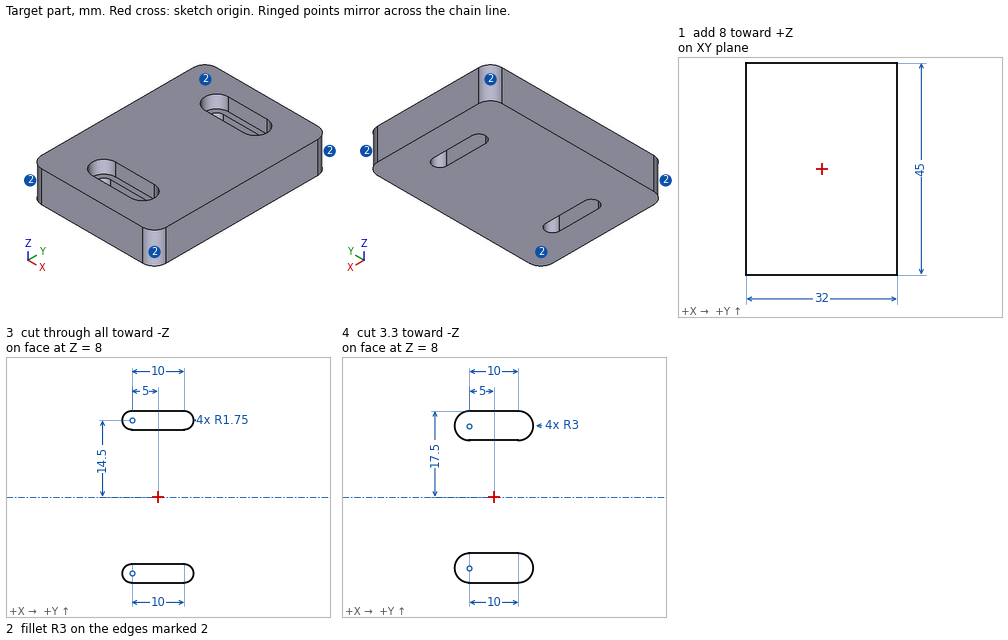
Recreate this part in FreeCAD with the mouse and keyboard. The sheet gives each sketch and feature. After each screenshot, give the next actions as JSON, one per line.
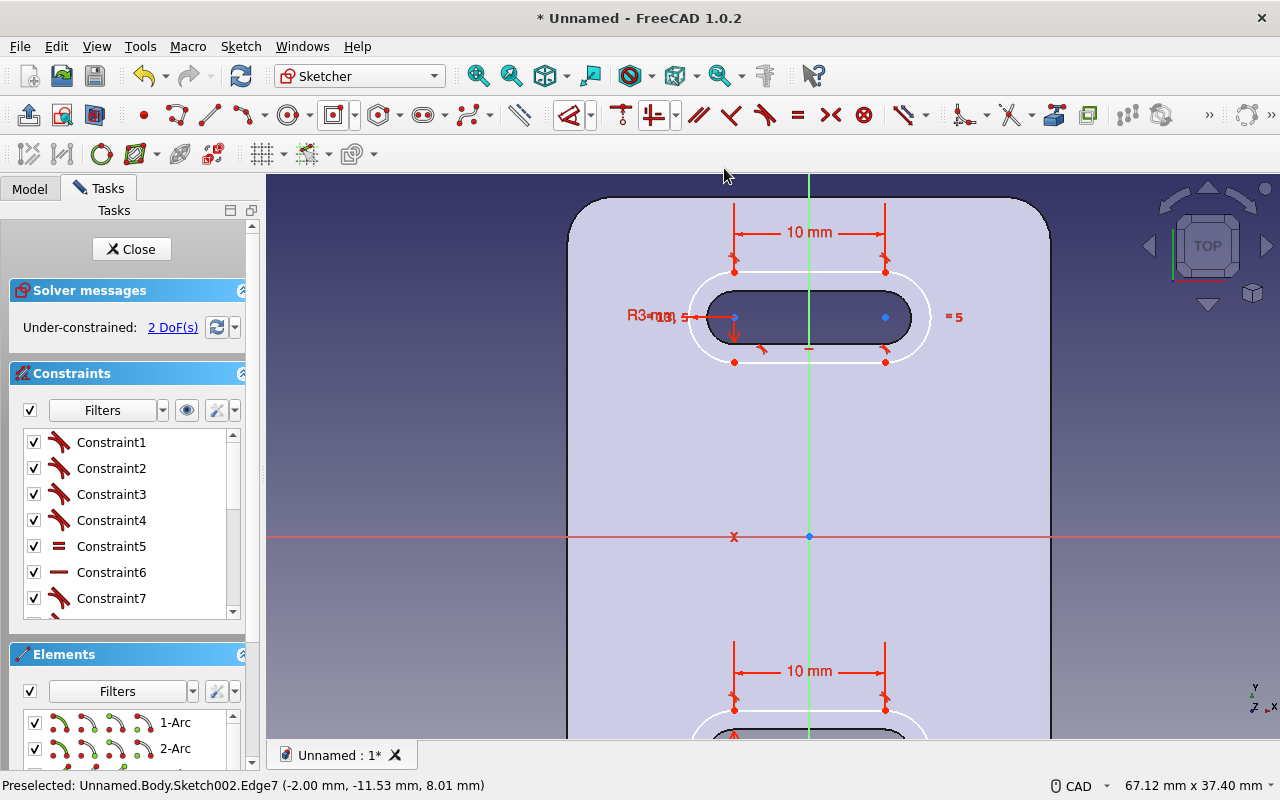
{"action": "left_click", "coordinate": [734, 272]}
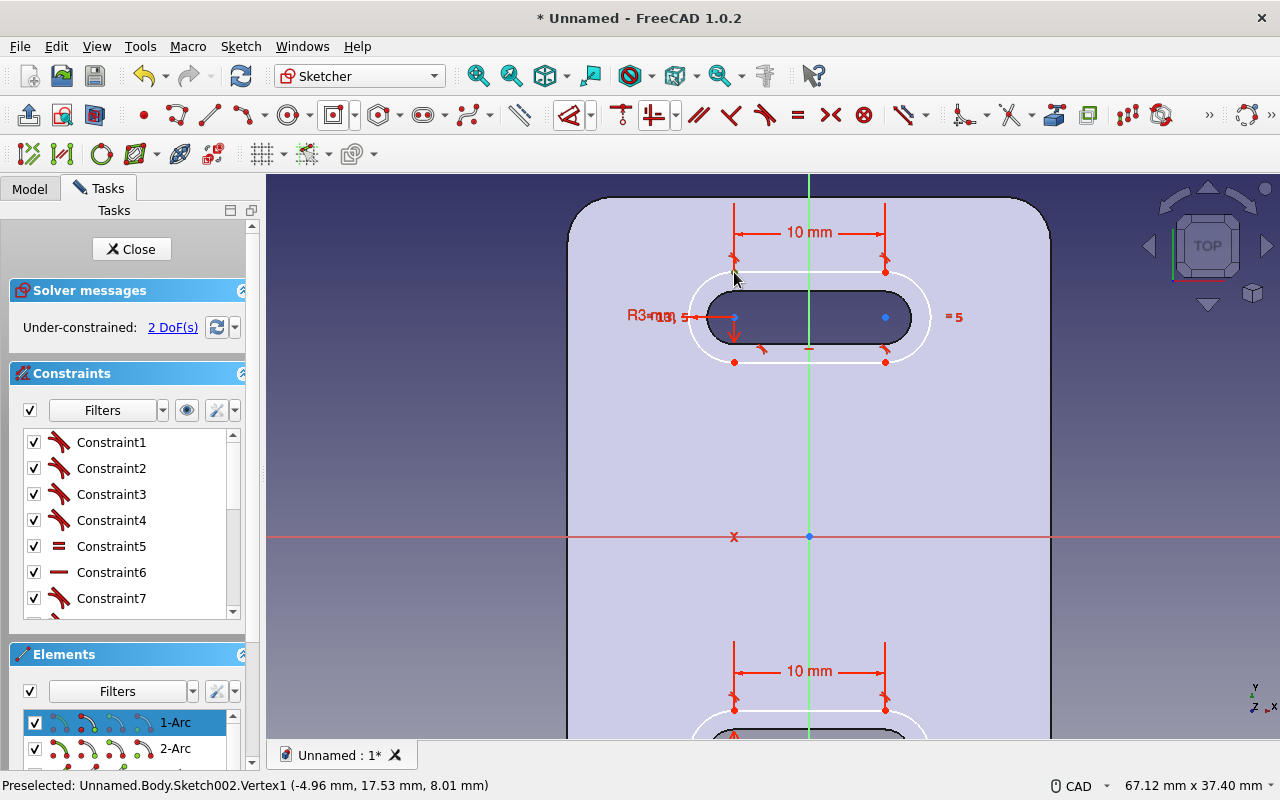
{"action": "key", "text": "l"}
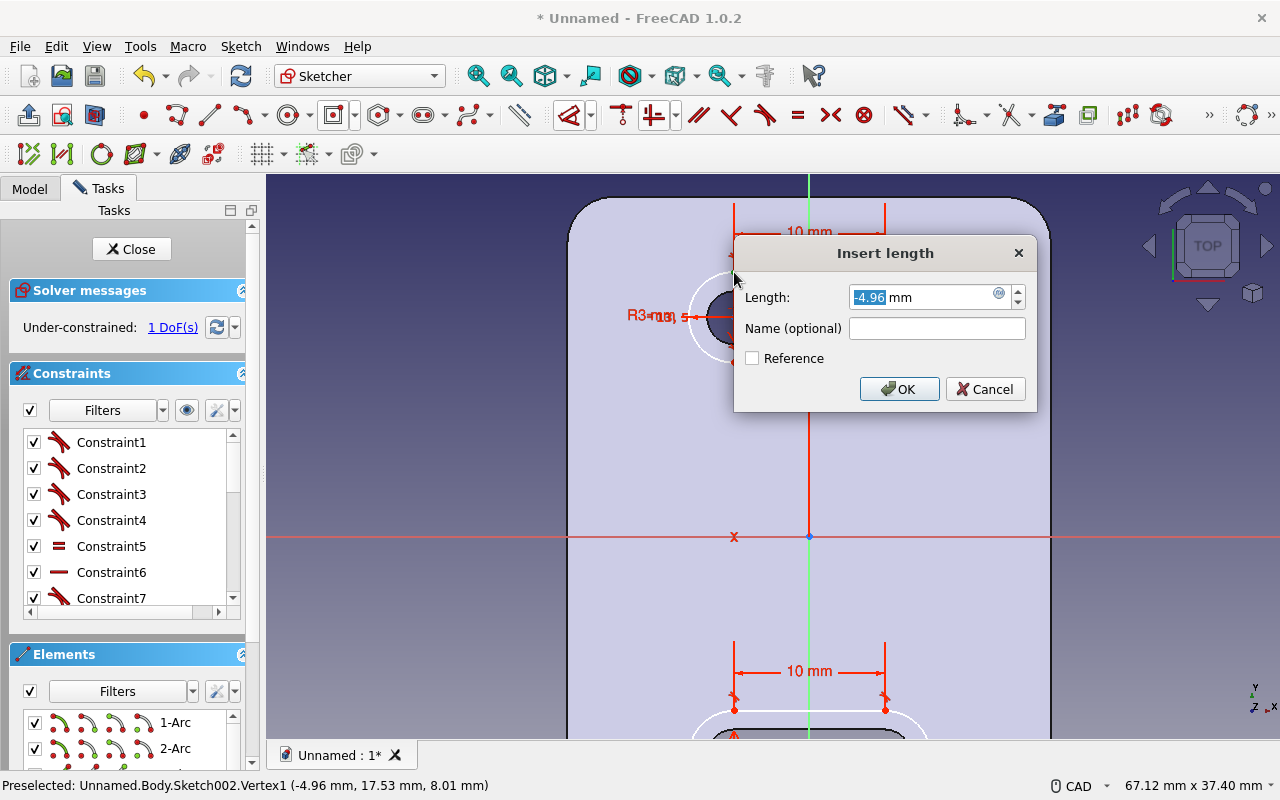
{"action": "type", "text": "-5"}
{"action": "key", "text": "Return"}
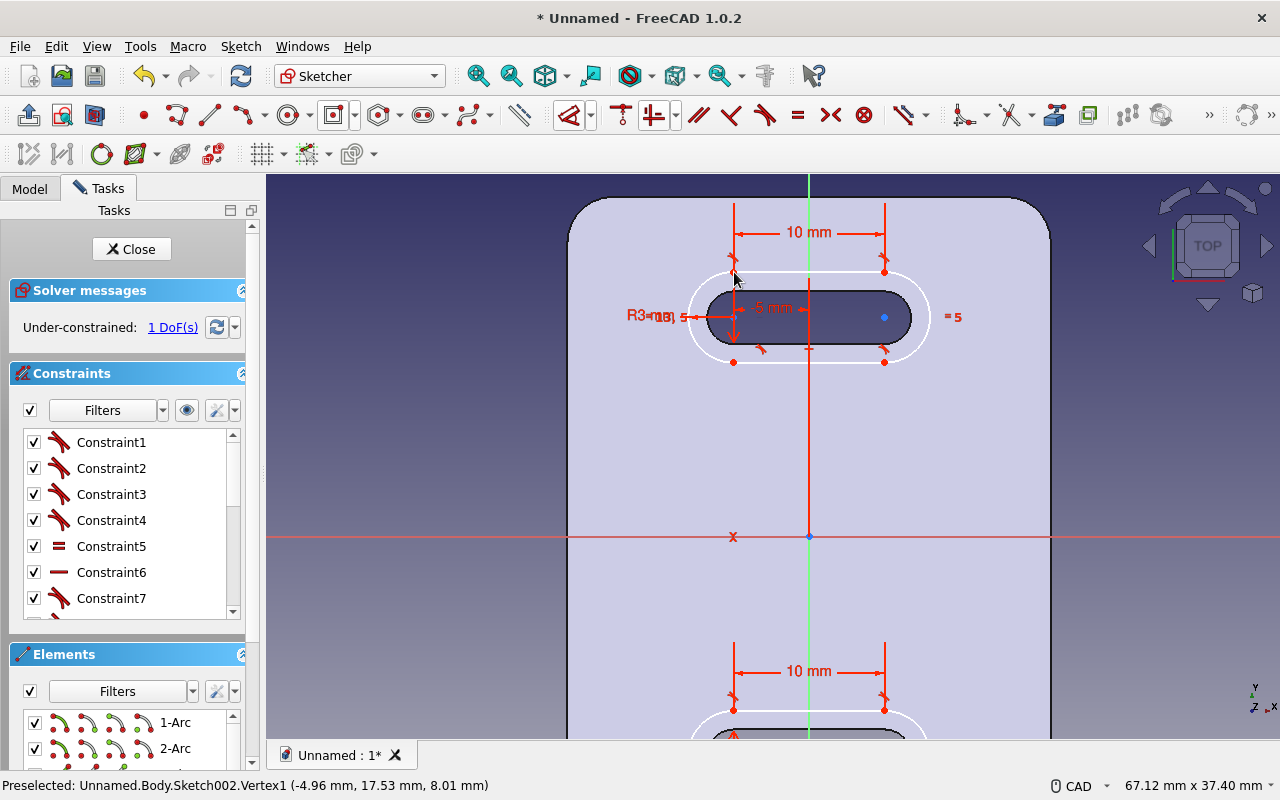
{"action": "left_click", "coordinate": [734, 272]}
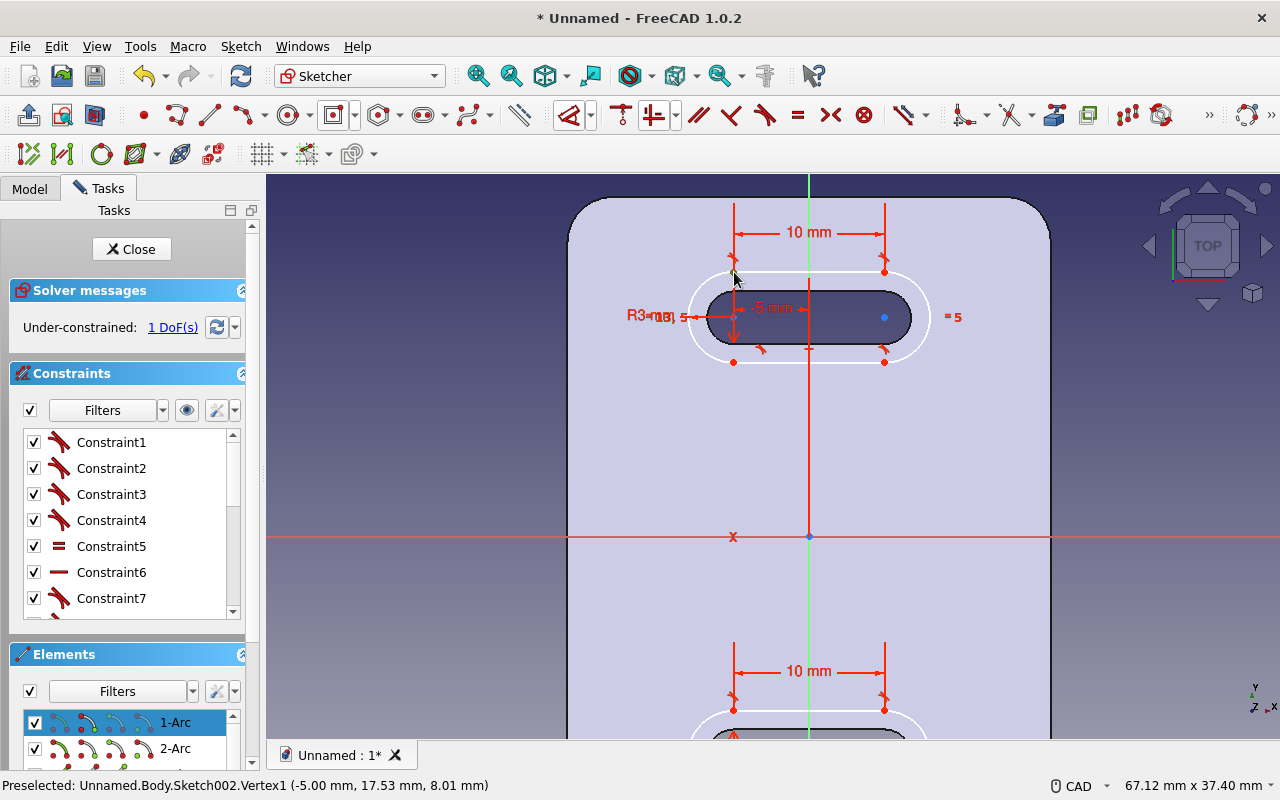
{"action": "key", "text": "i"}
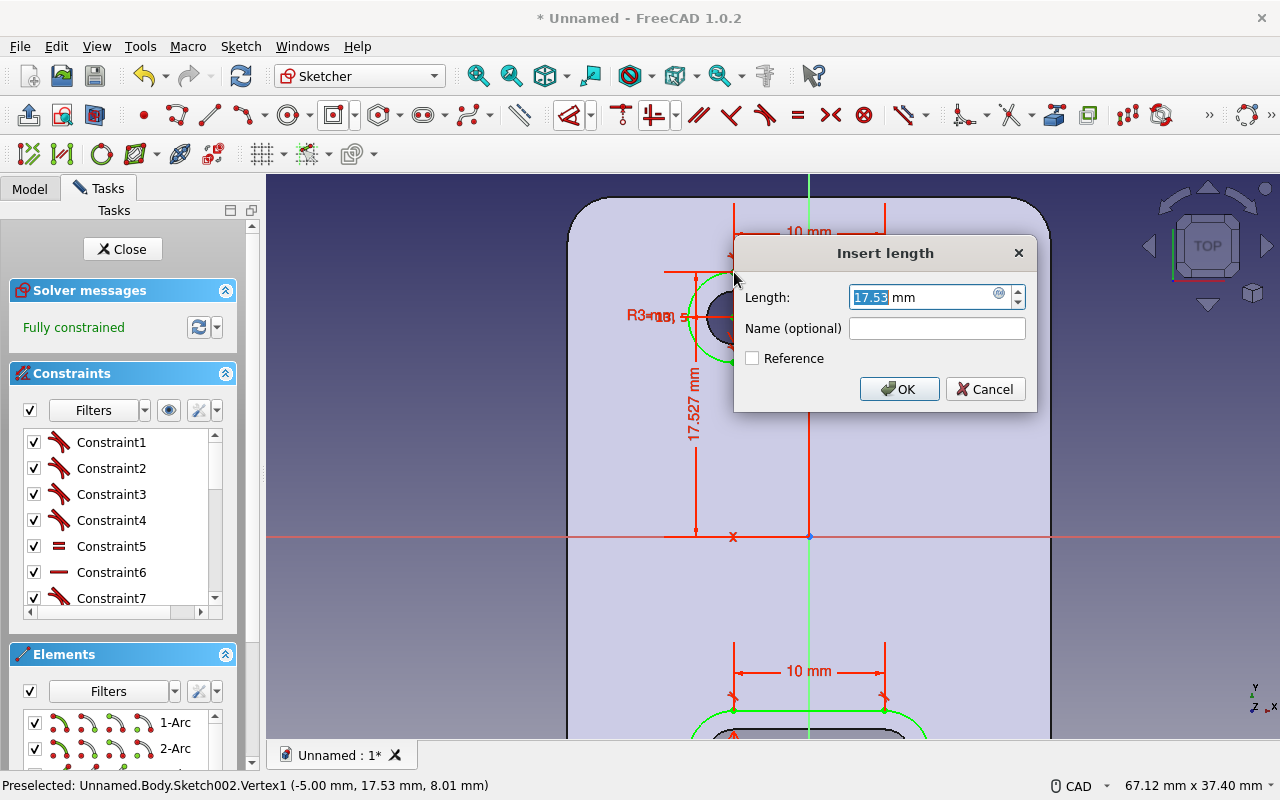
{"action": "type", "text": "17.5"}
{"action": "key", "text": "Return"}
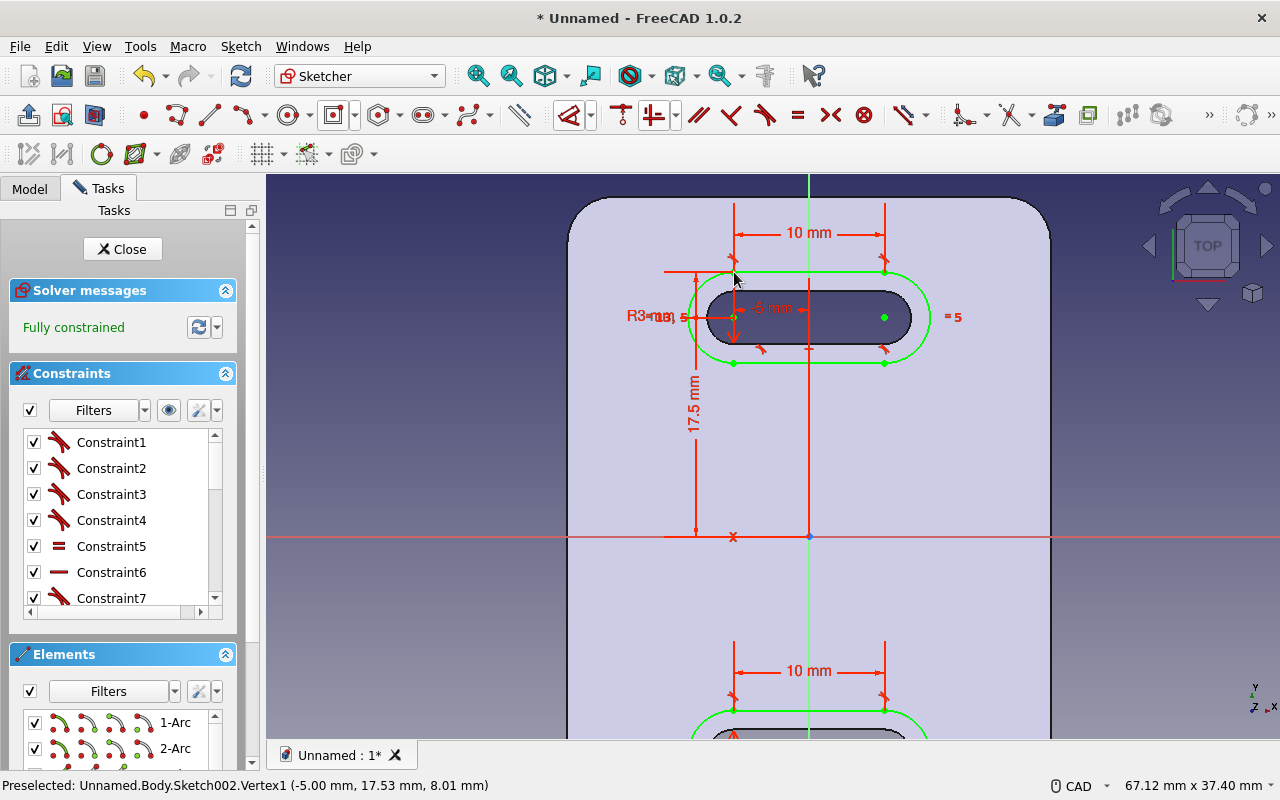
{"action": "left_click", "coordinate": [123, 249]}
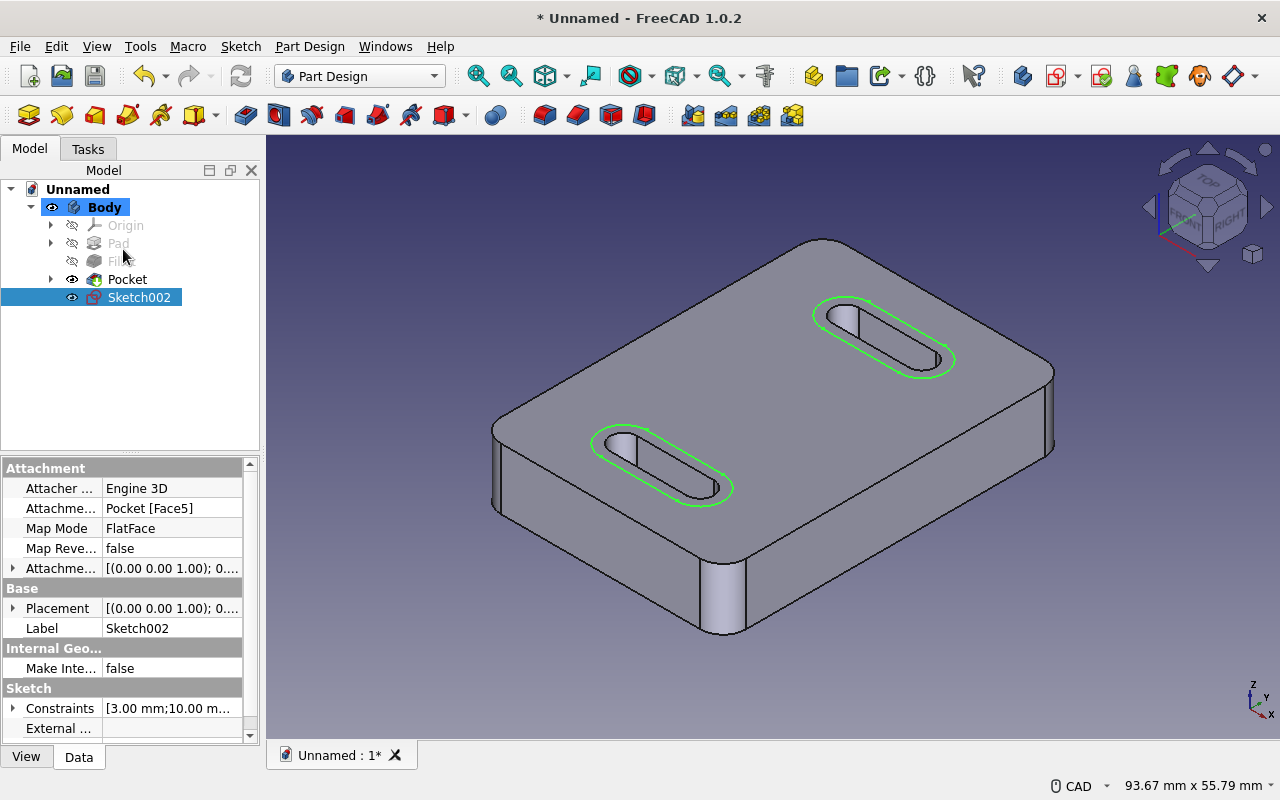
{"action": "left_click", "coordinate": [246, 116]}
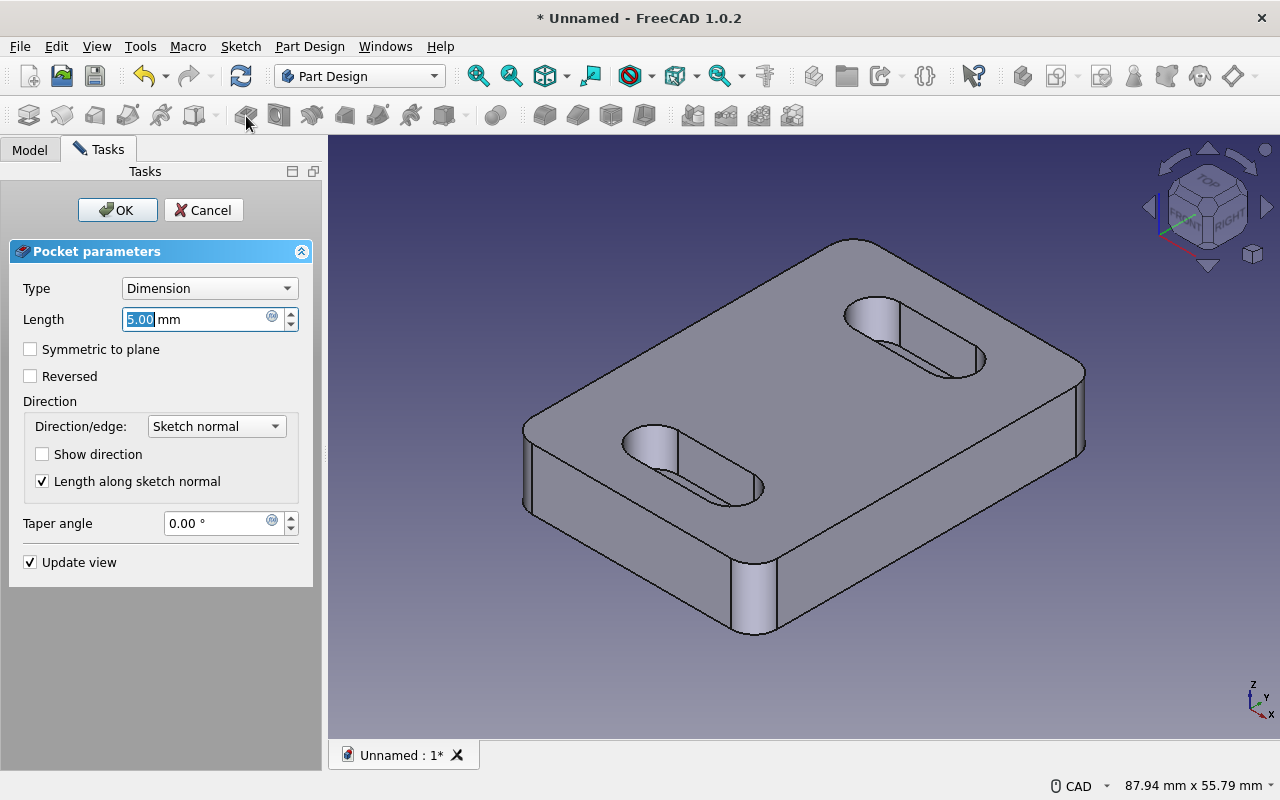
{"action": "type", "text": "3.3"}
{"action": "key", "text": "Tab"}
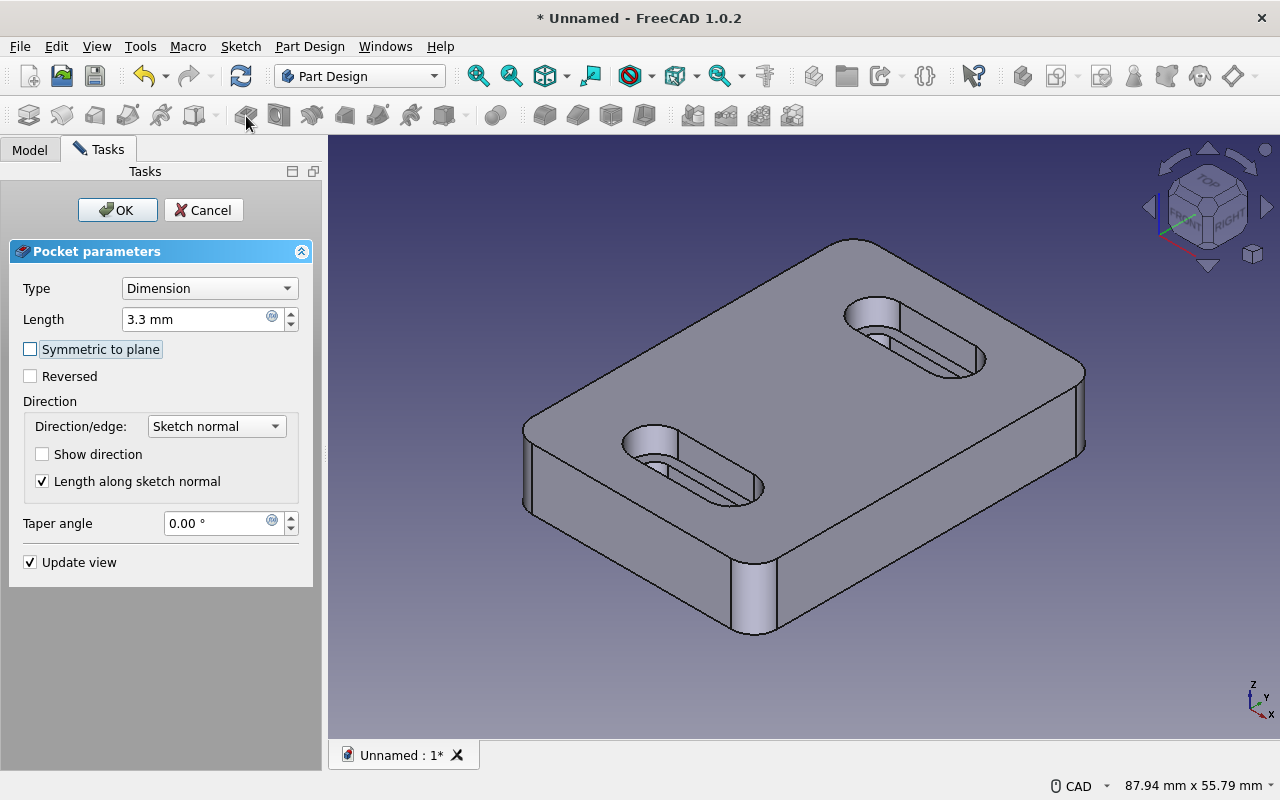
{"action": "left_click", "coordinate": [118, 210]}